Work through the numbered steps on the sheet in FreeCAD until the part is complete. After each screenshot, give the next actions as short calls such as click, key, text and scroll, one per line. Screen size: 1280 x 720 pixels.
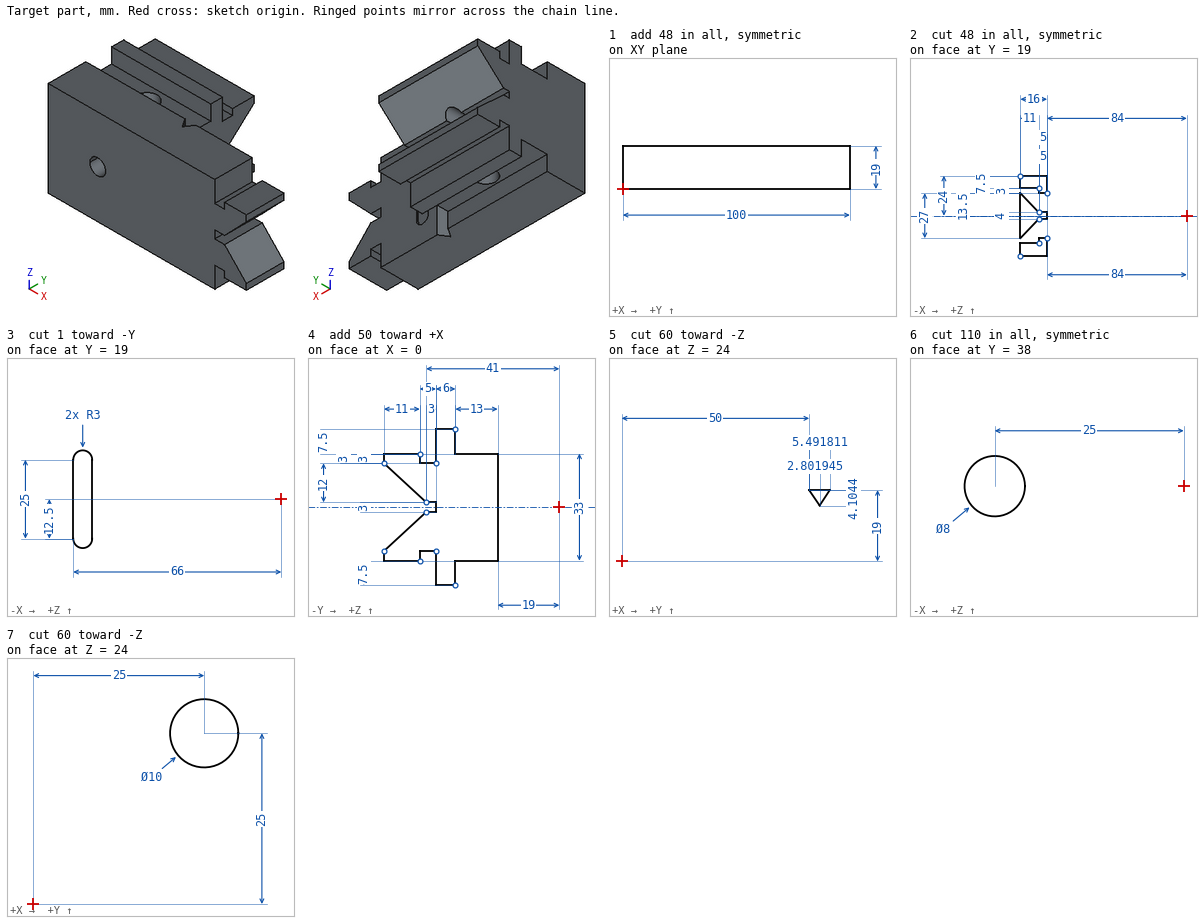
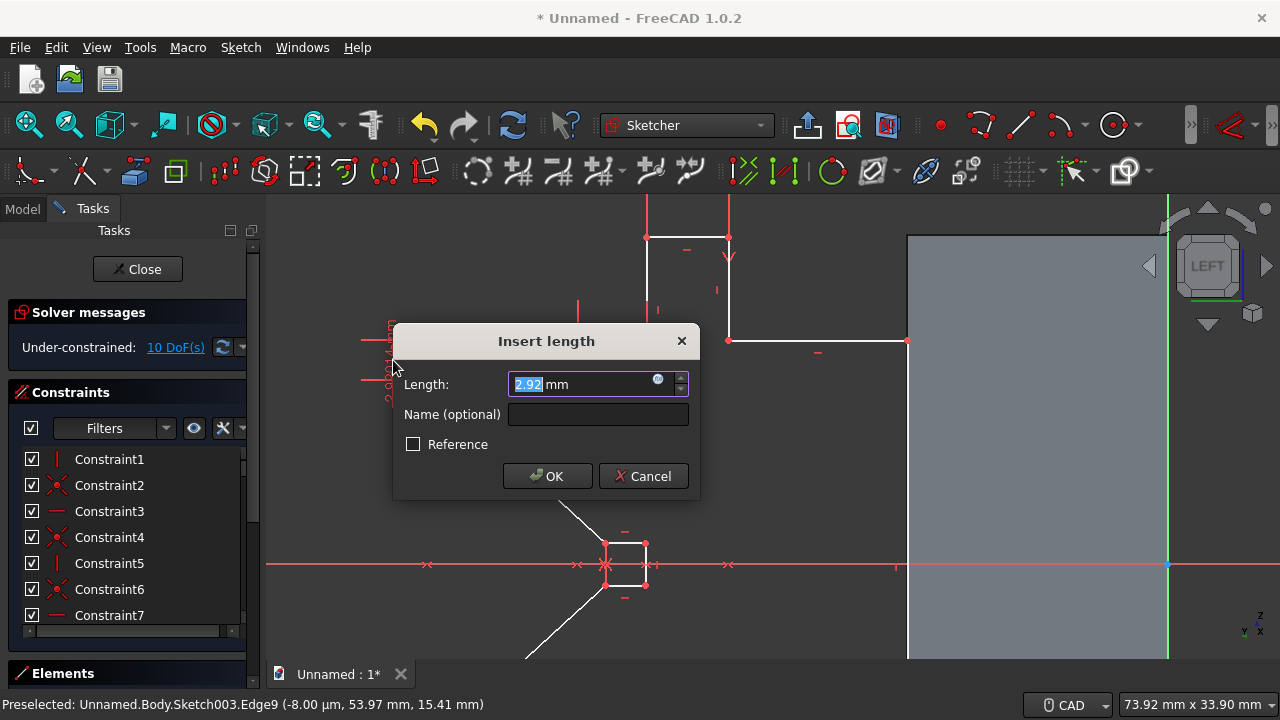
text(3)
key(Return)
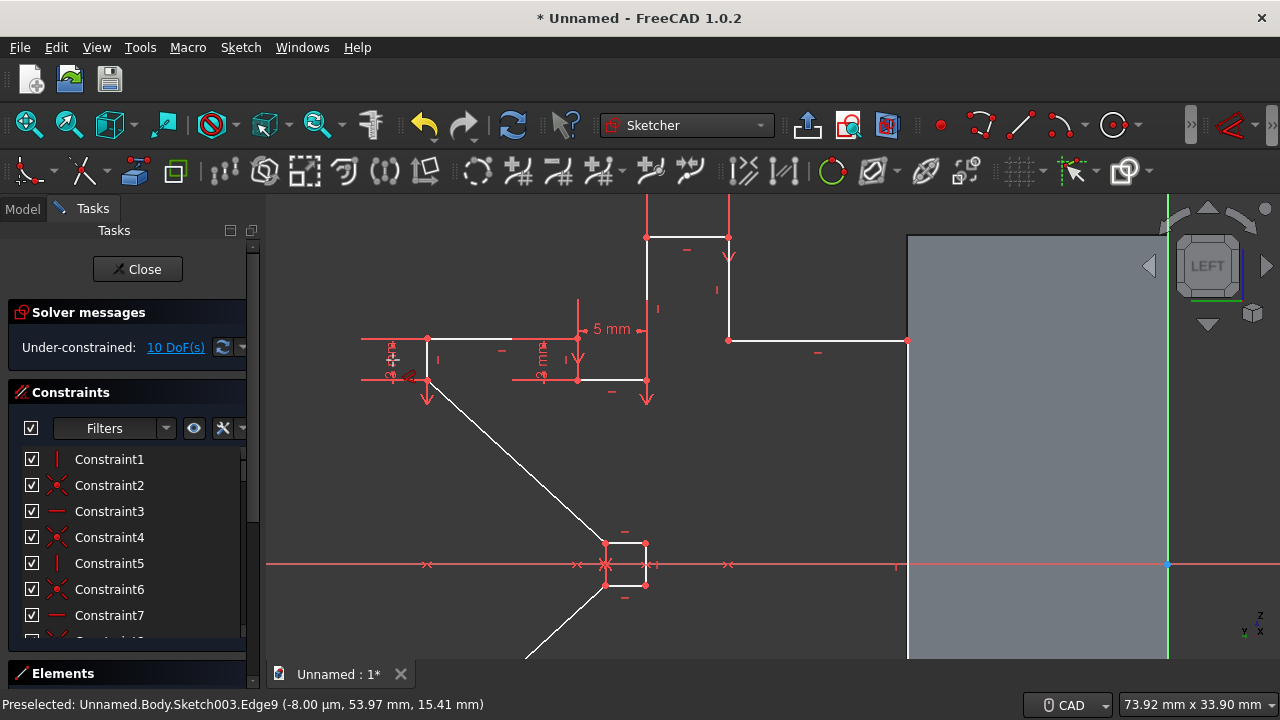
click(618, 543)
click(626, 509)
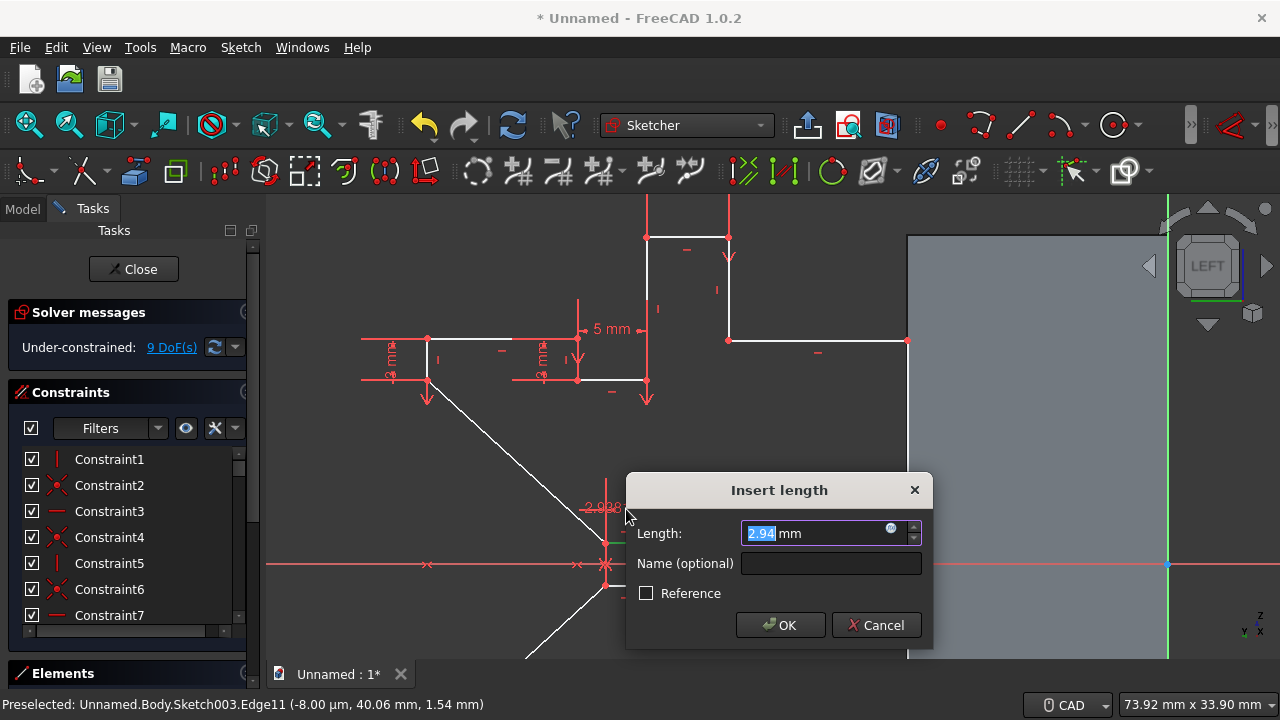
text(3)
key(Return)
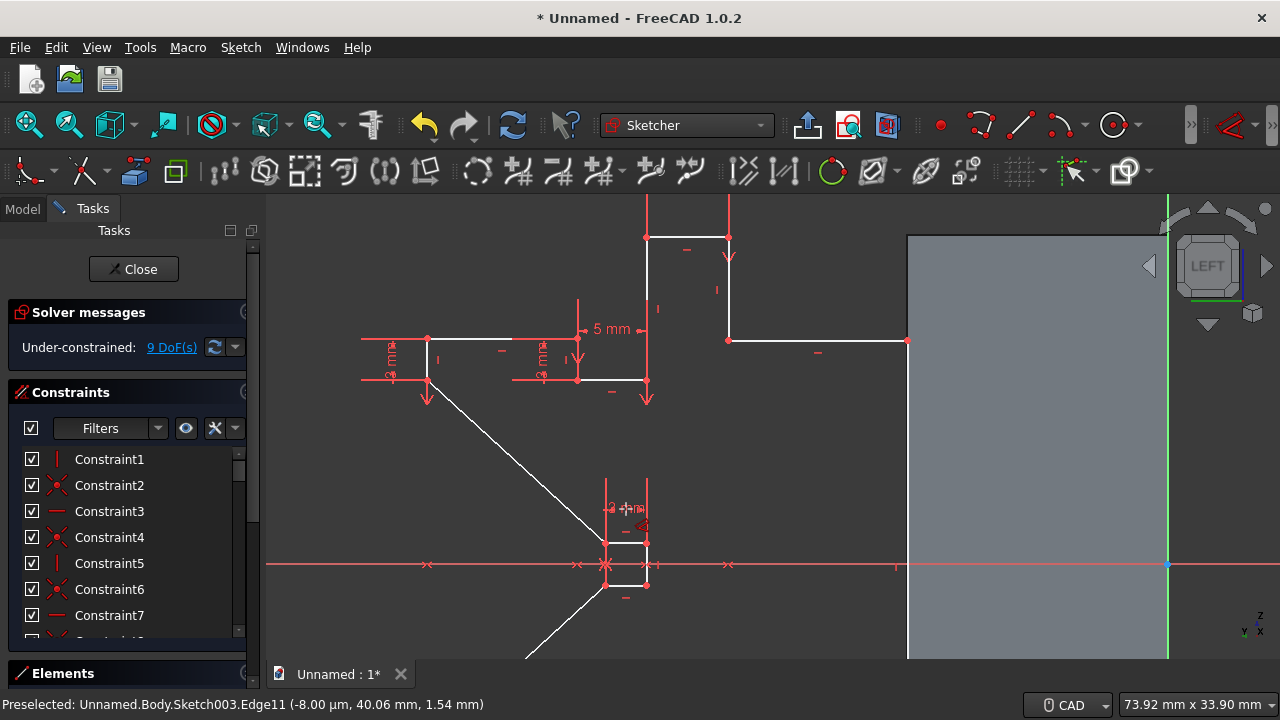
click(647, 564)
click(681, 550)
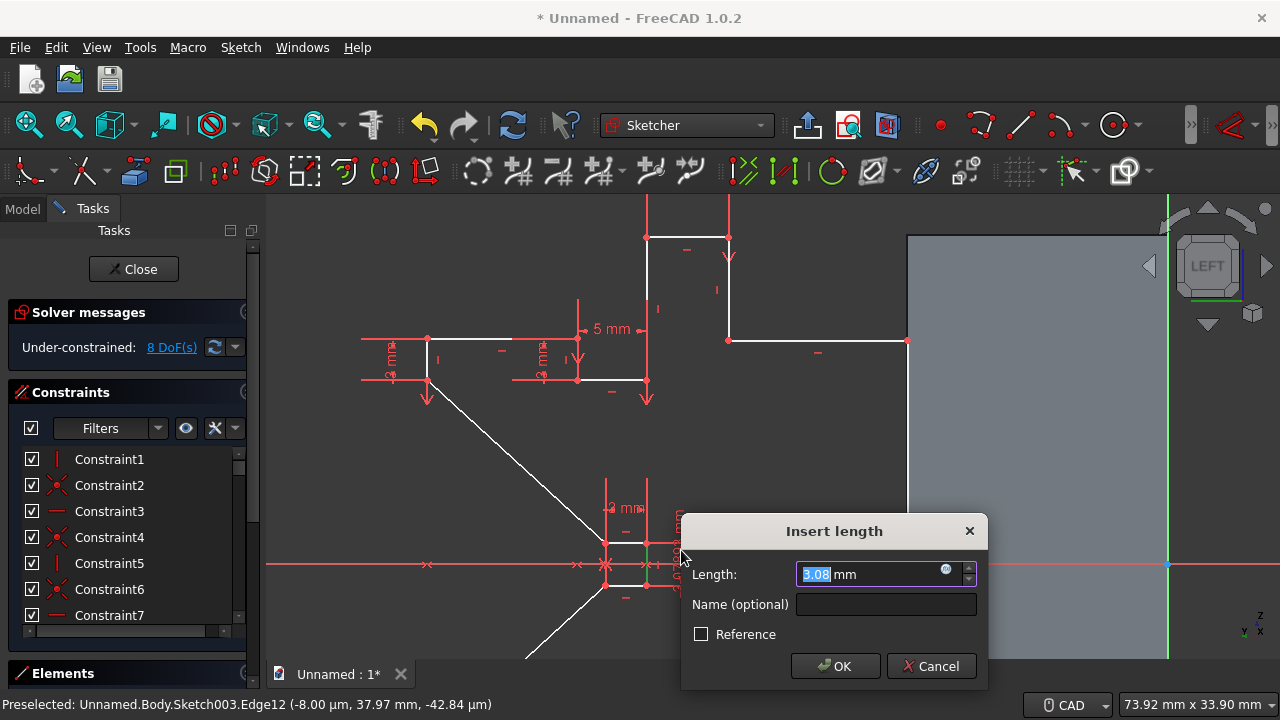
text(3)
key(Return)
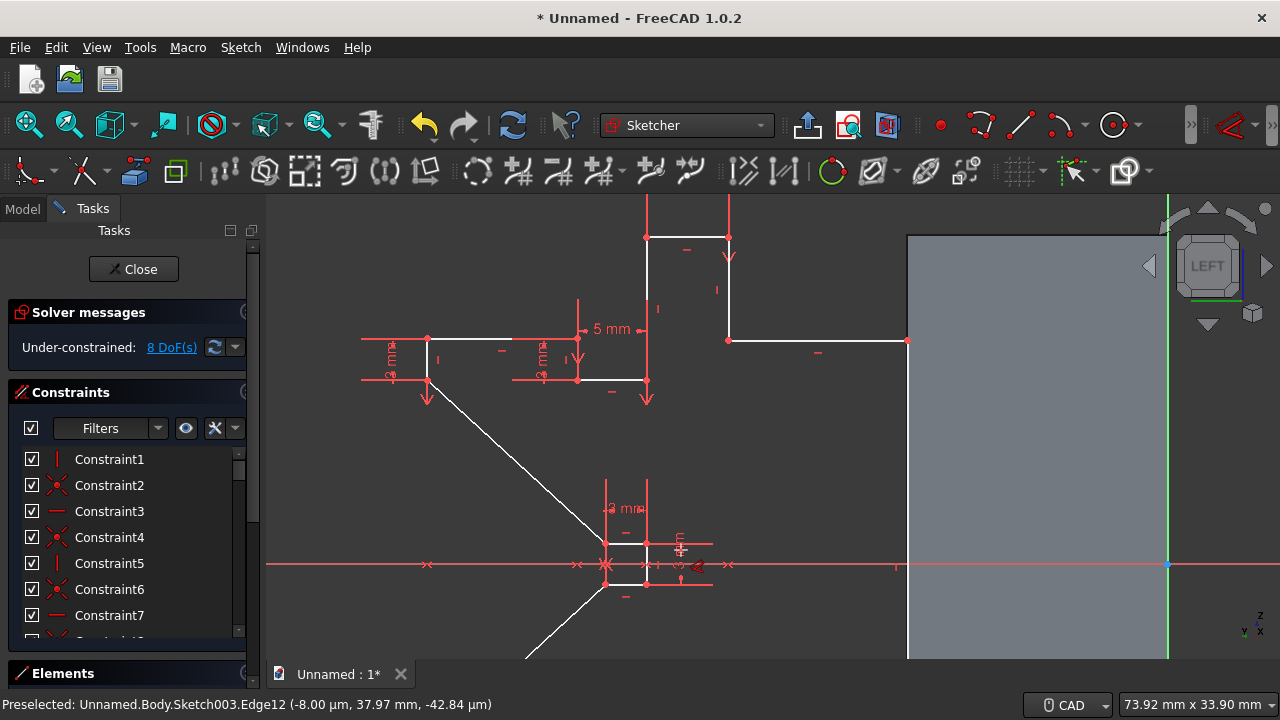
click(908, 476)
click(942, 486)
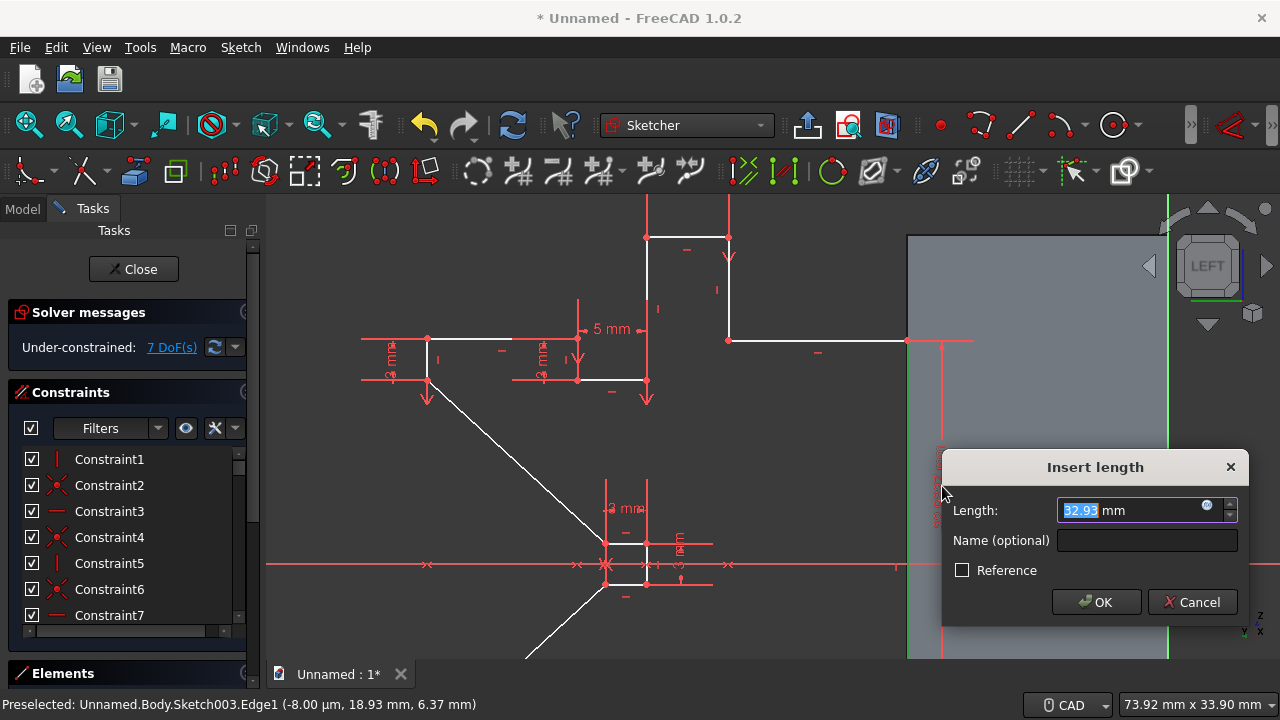
text(33)
key(Return)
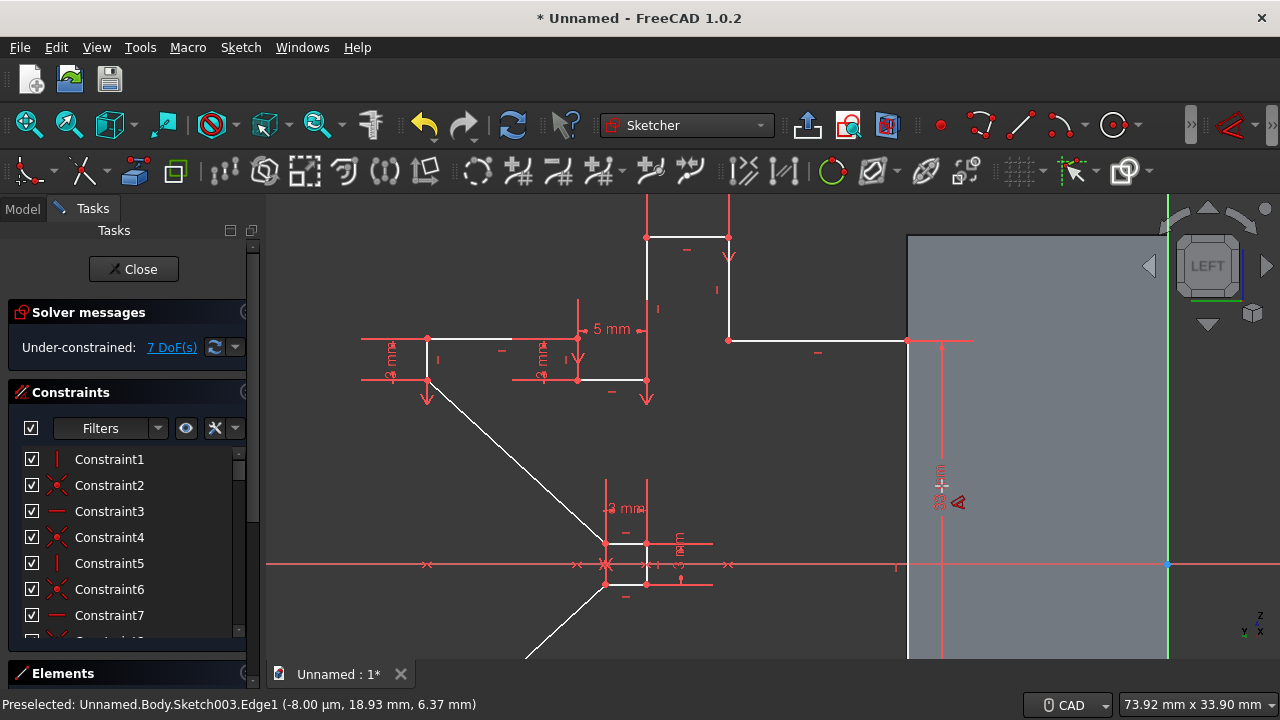
click(854, 341)
click(818, 307)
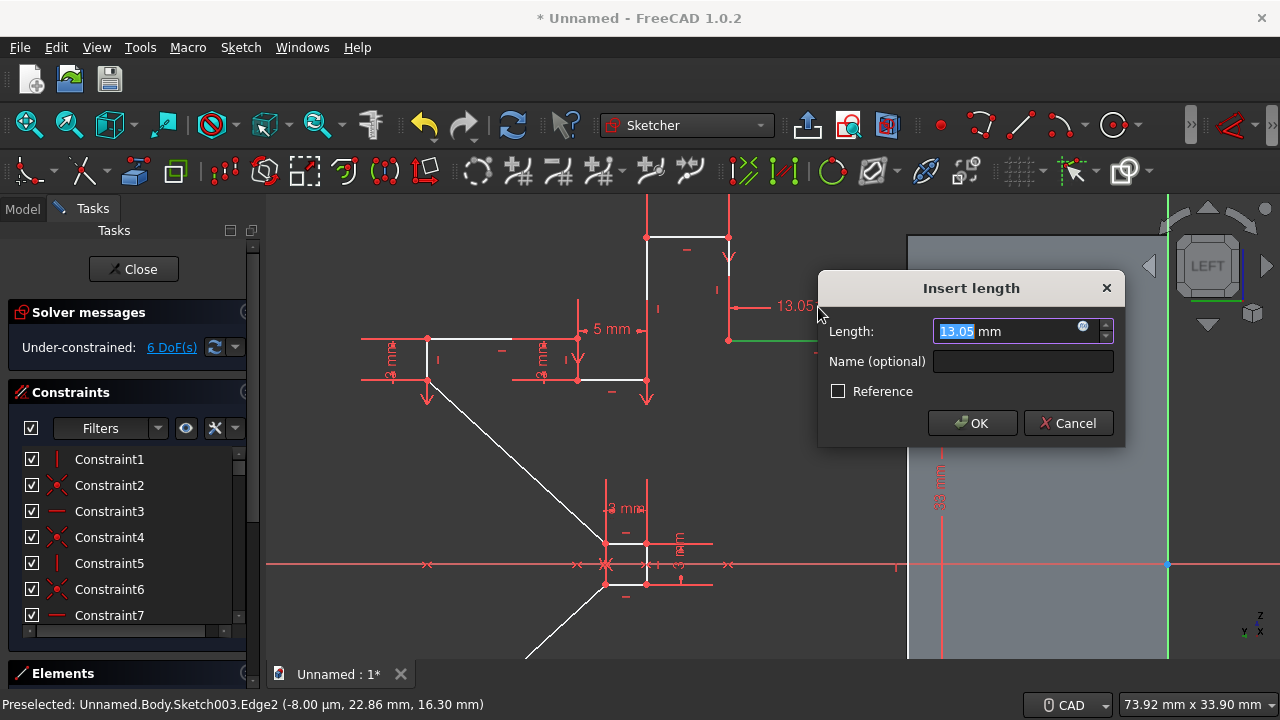
text(13)
key(Return)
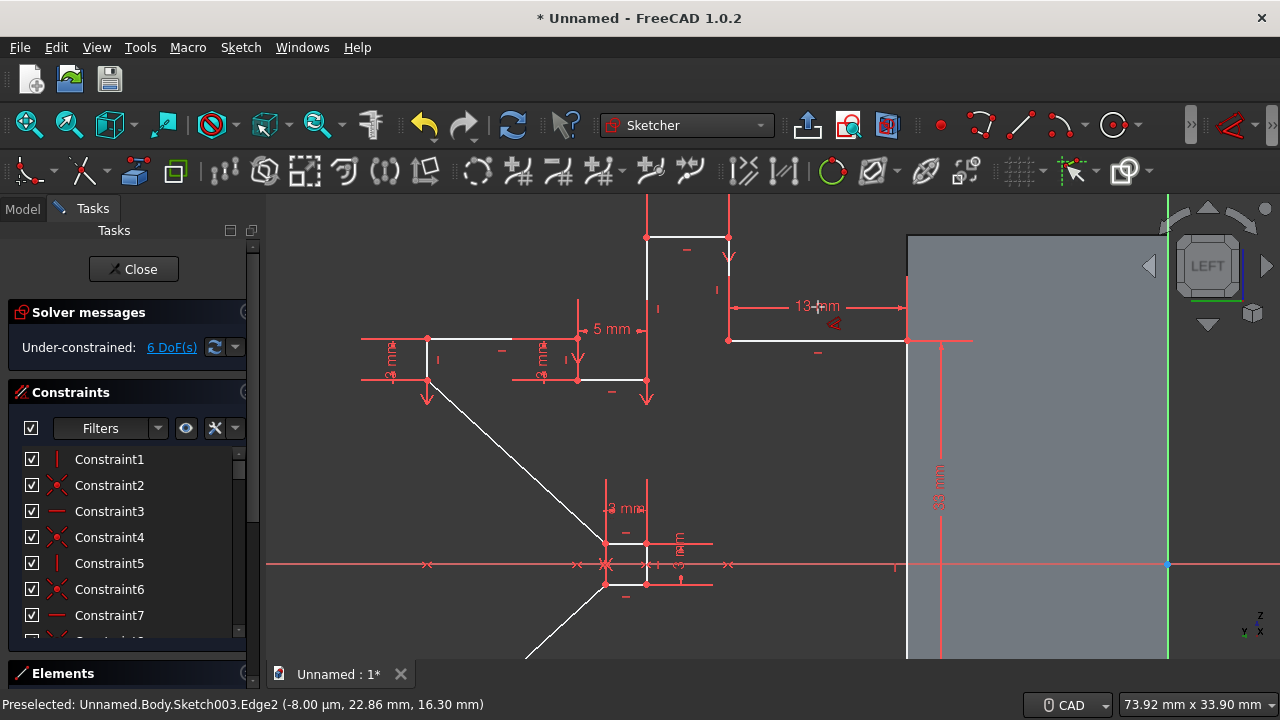
click(533, 339)
click(503, 305)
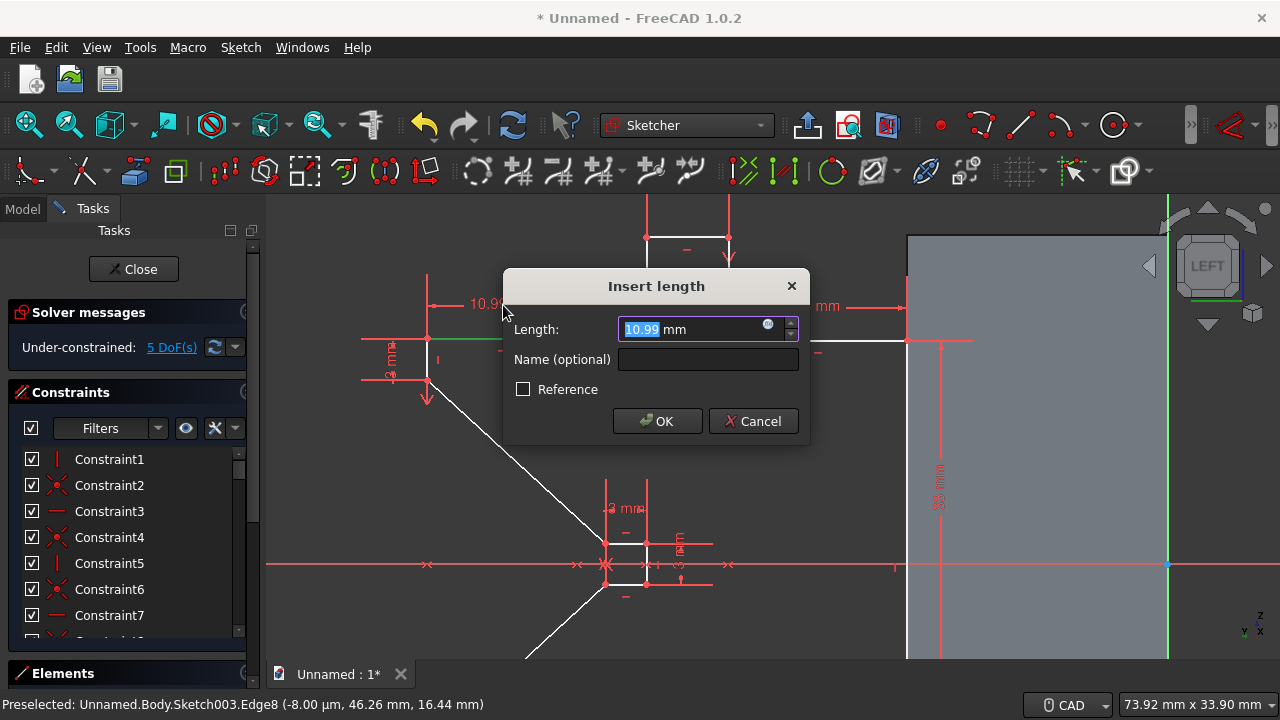
text(11)
key(Return)